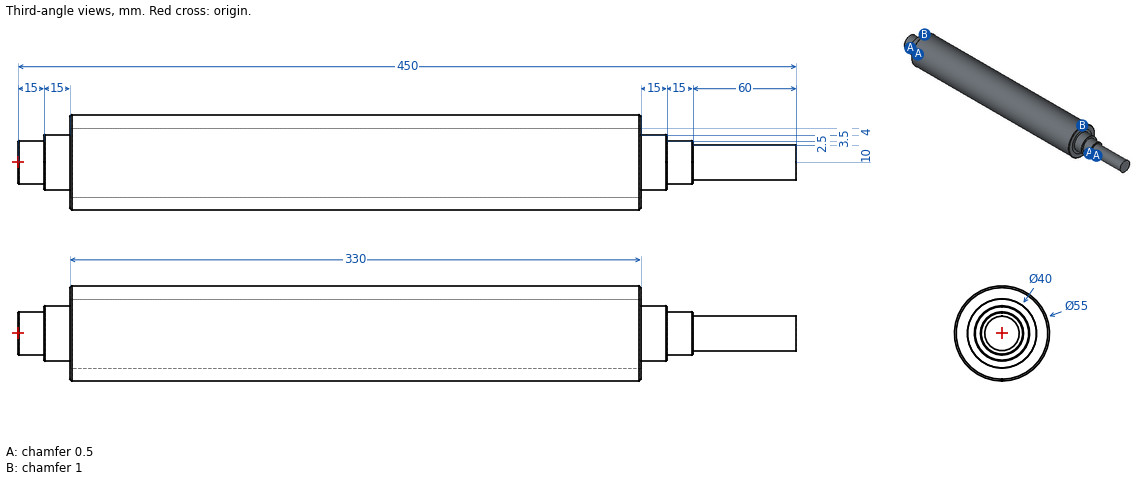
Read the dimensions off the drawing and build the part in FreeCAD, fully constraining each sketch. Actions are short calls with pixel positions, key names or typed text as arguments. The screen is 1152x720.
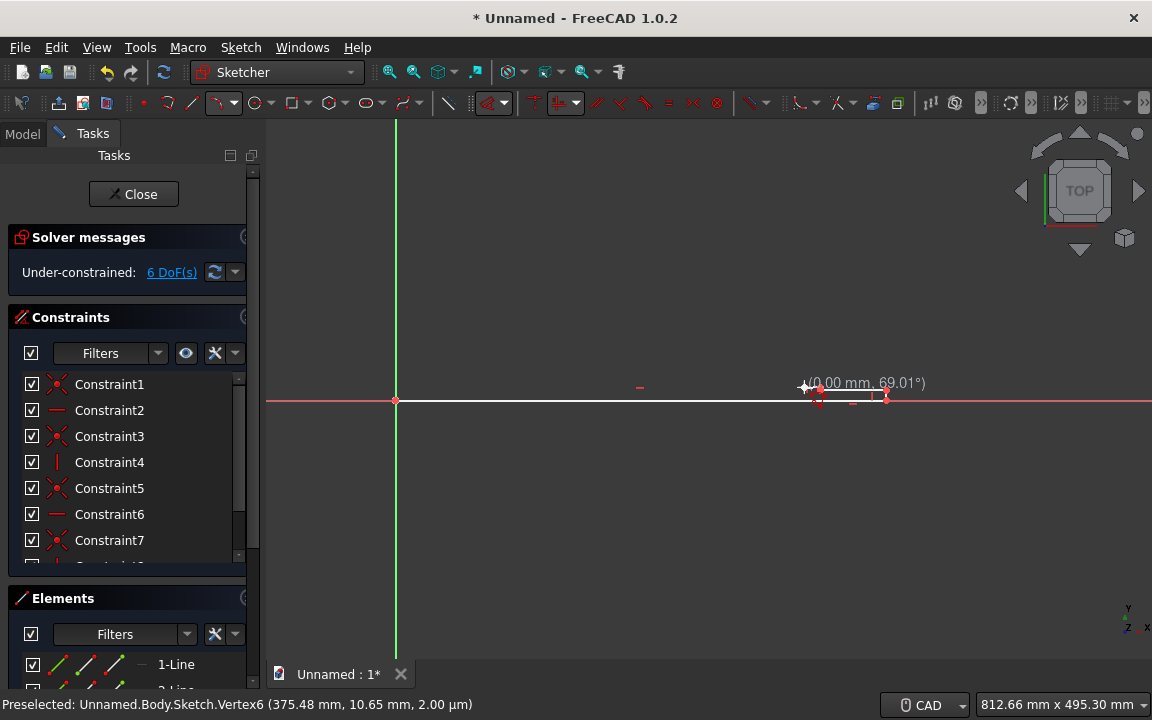
scroll(804, 383, up, 8)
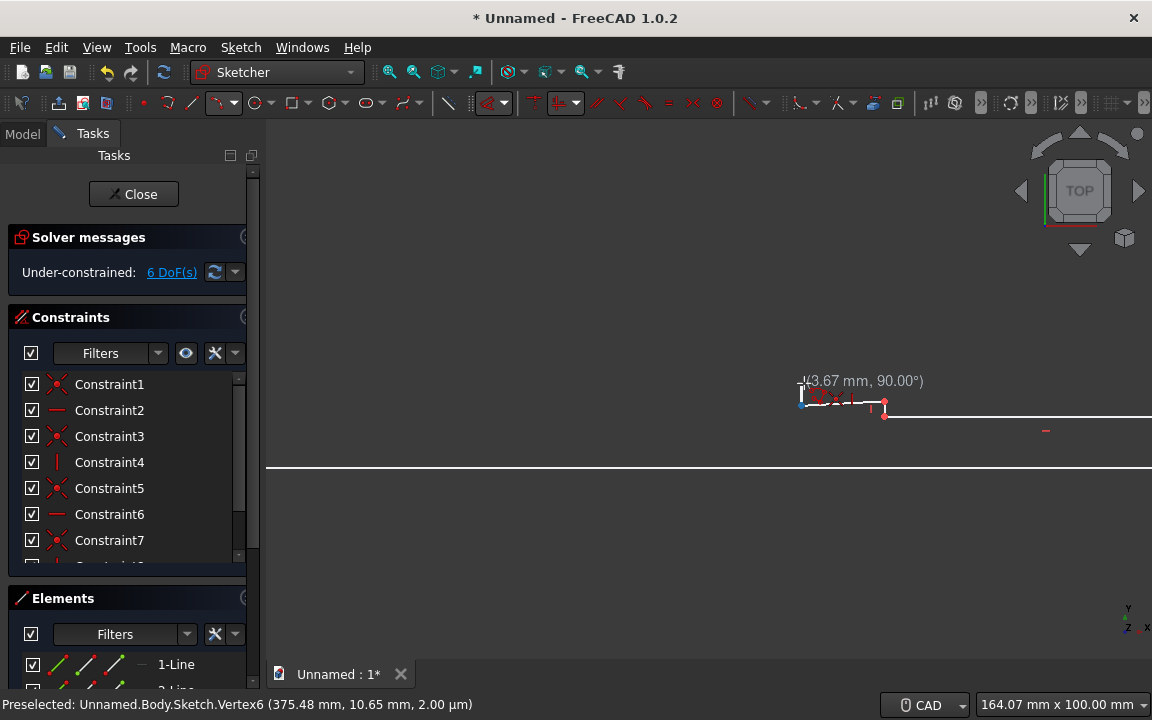
click(802, 382)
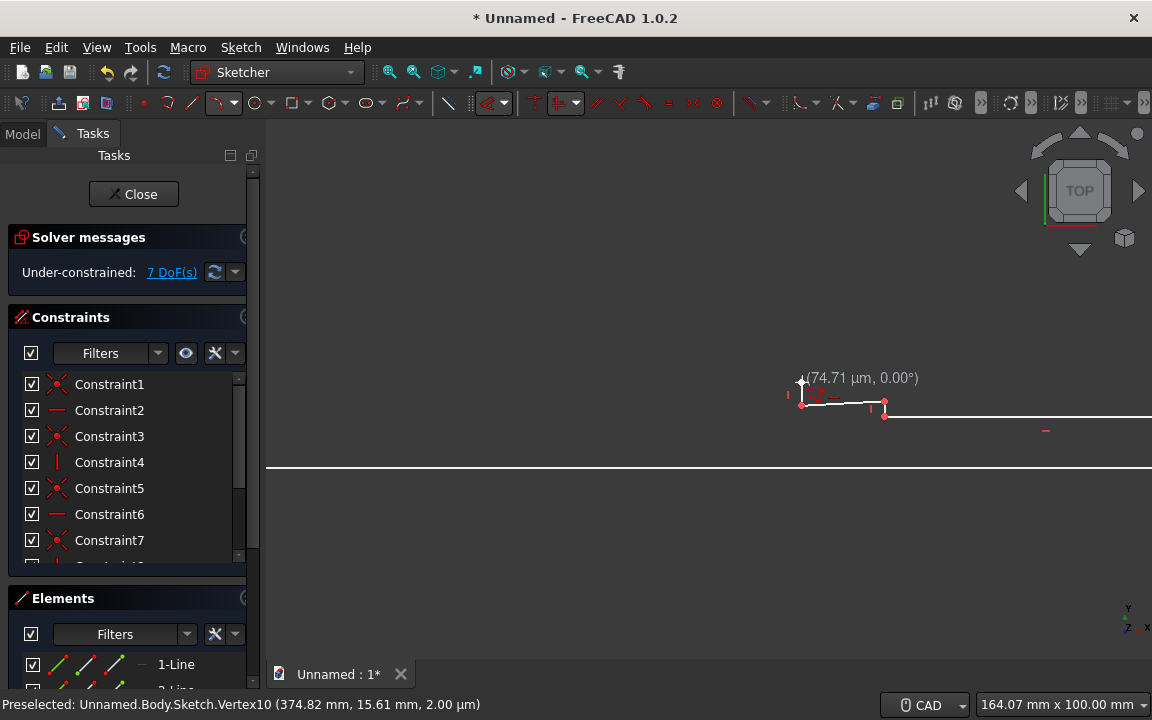
scroll(804, 383, down, 8)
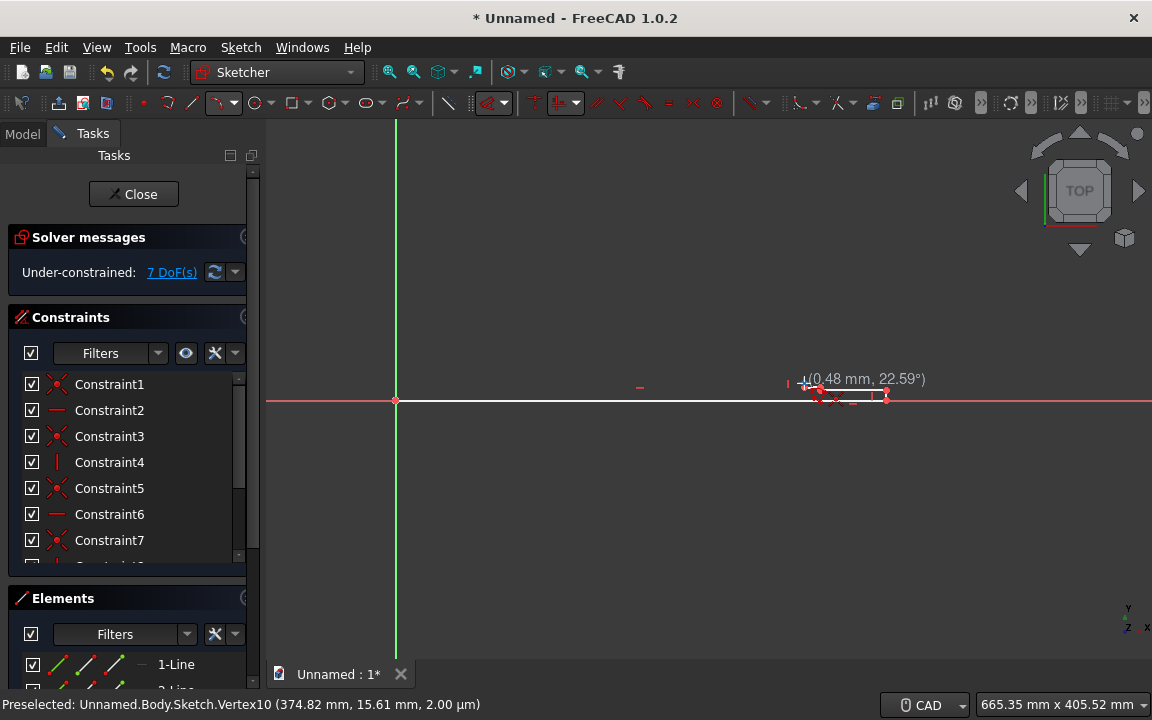
click(788, 383)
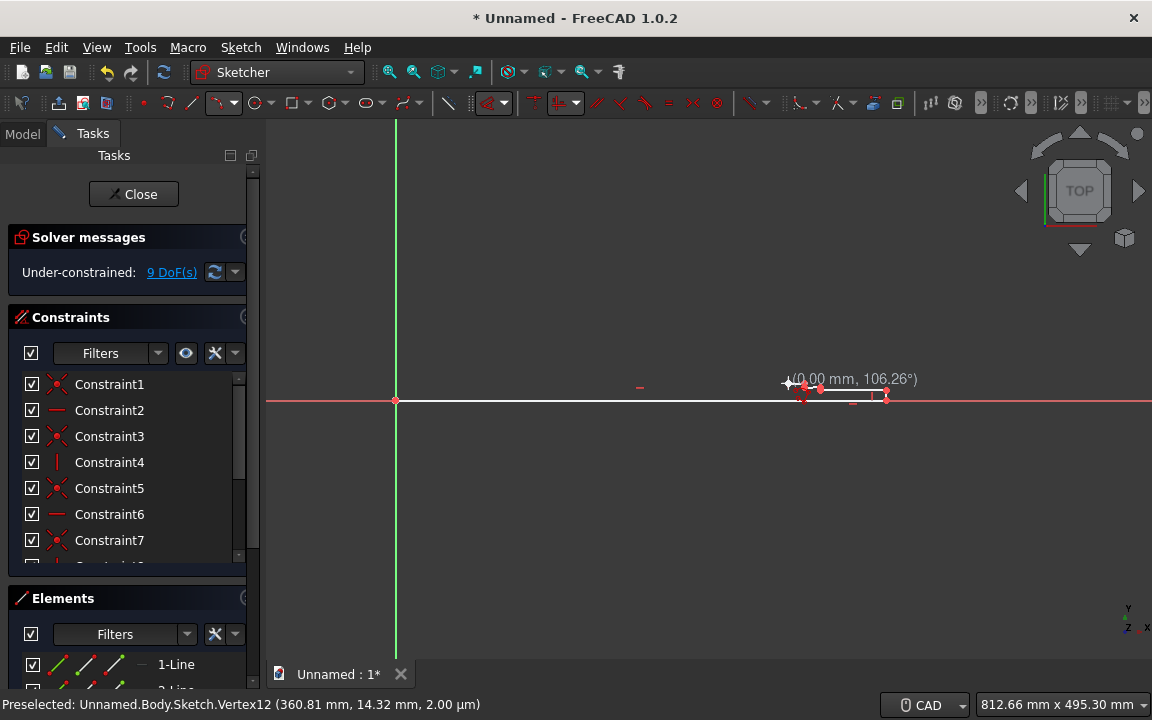
scroll(788, 379, up, 7)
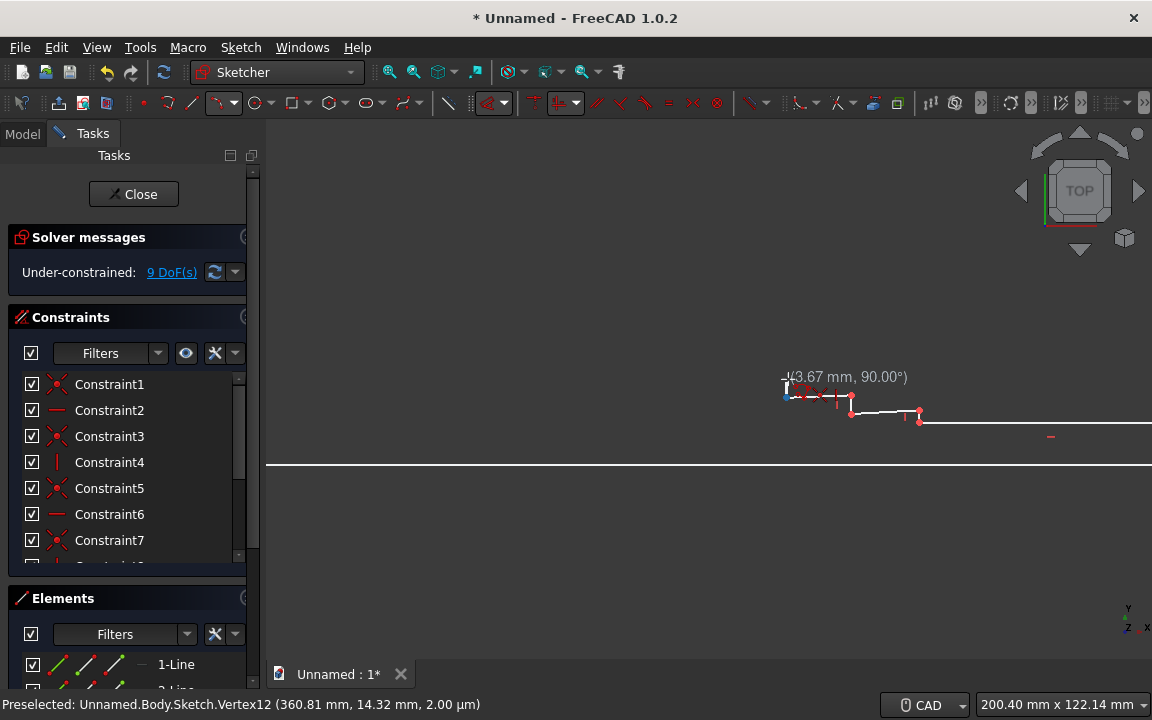
click(786, 377)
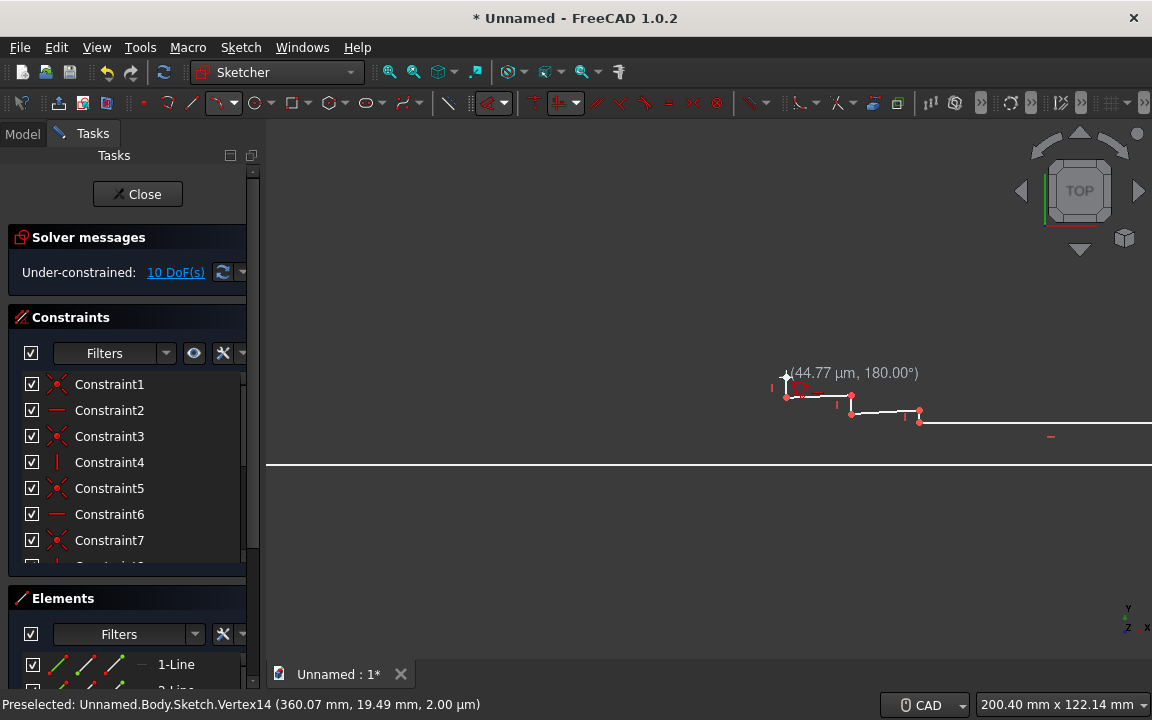
scroll(788, 379, down, 7)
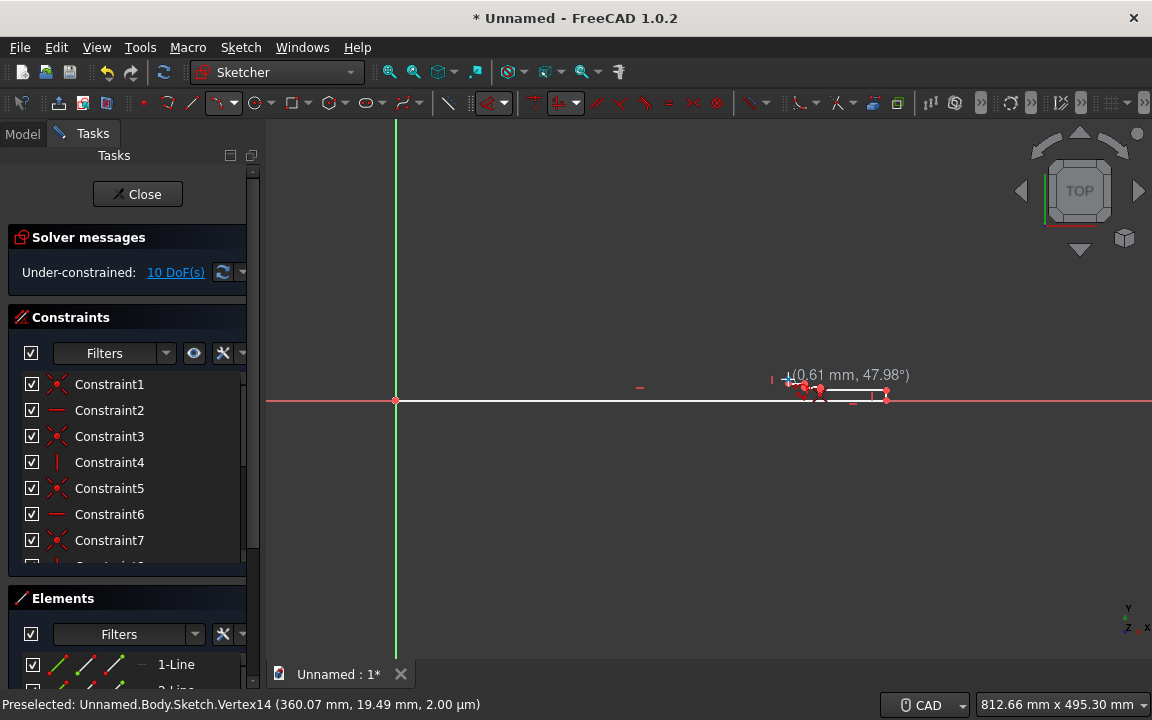
click(428, 379)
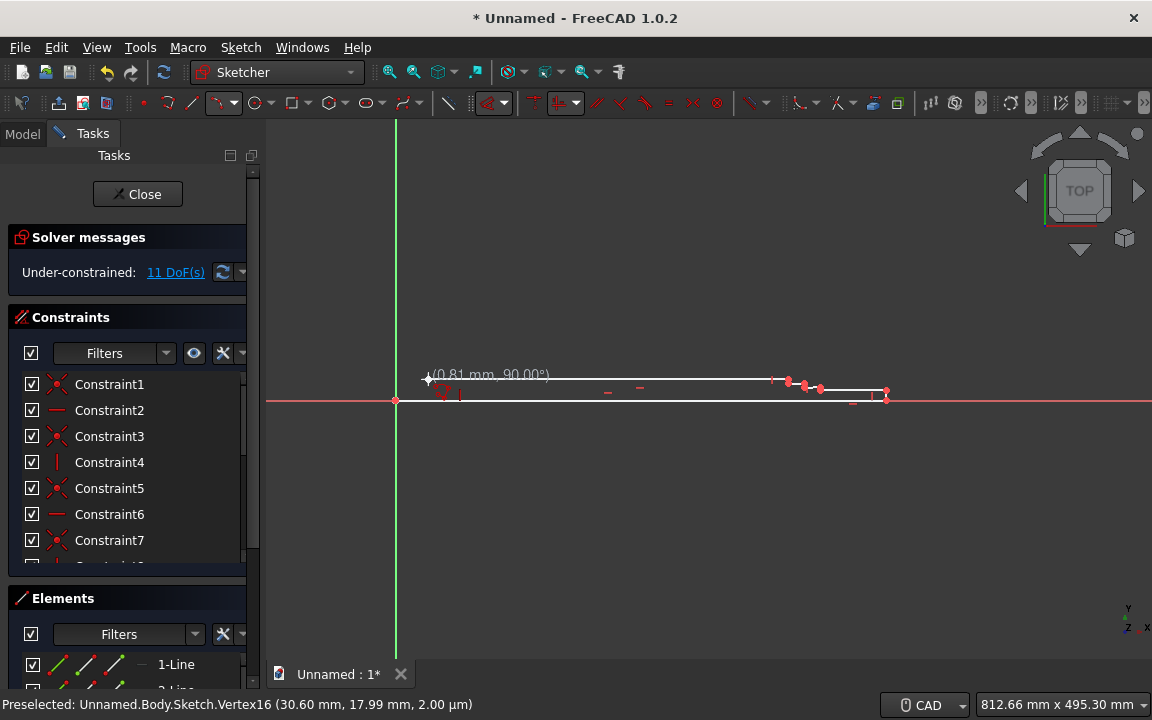
scroll(428, 383, up, 7)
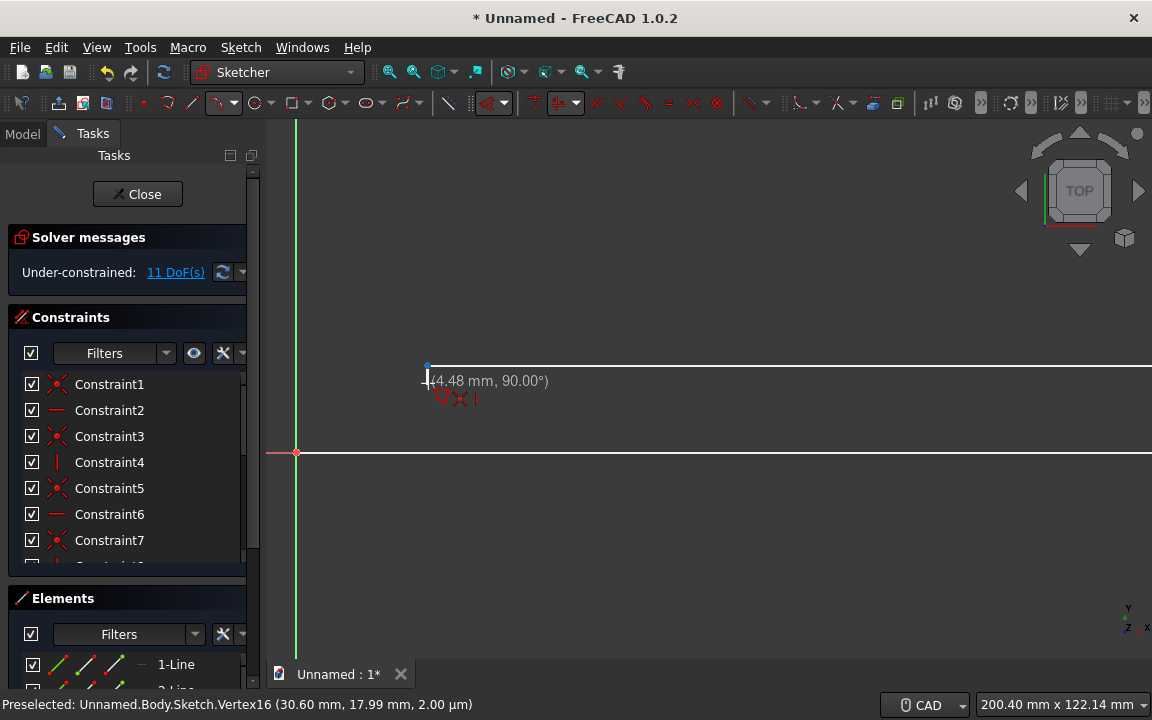
click(427, 382)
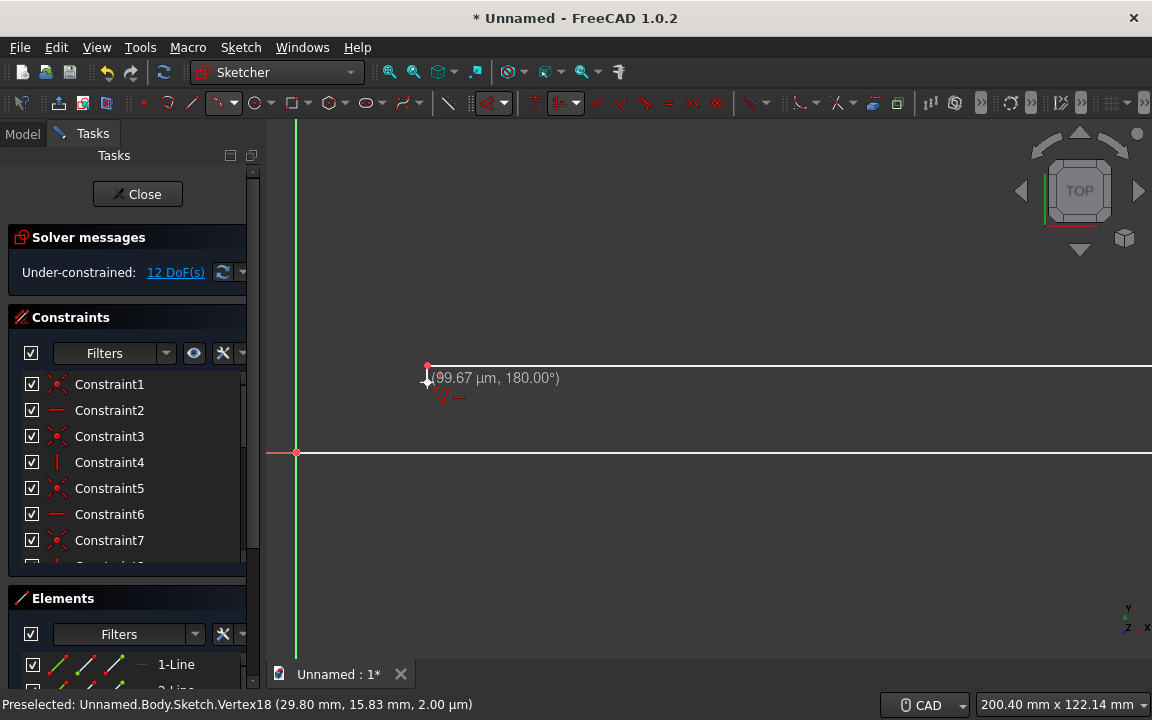
scroll(428, 383, down, 7)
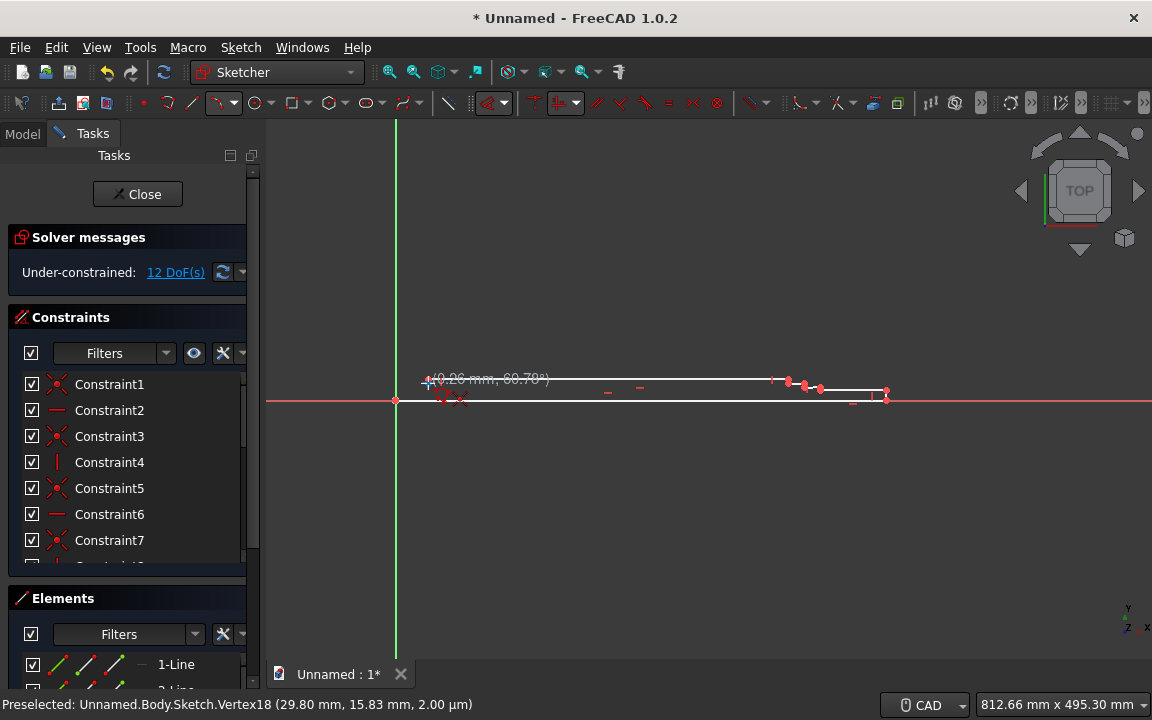
click(412, 383)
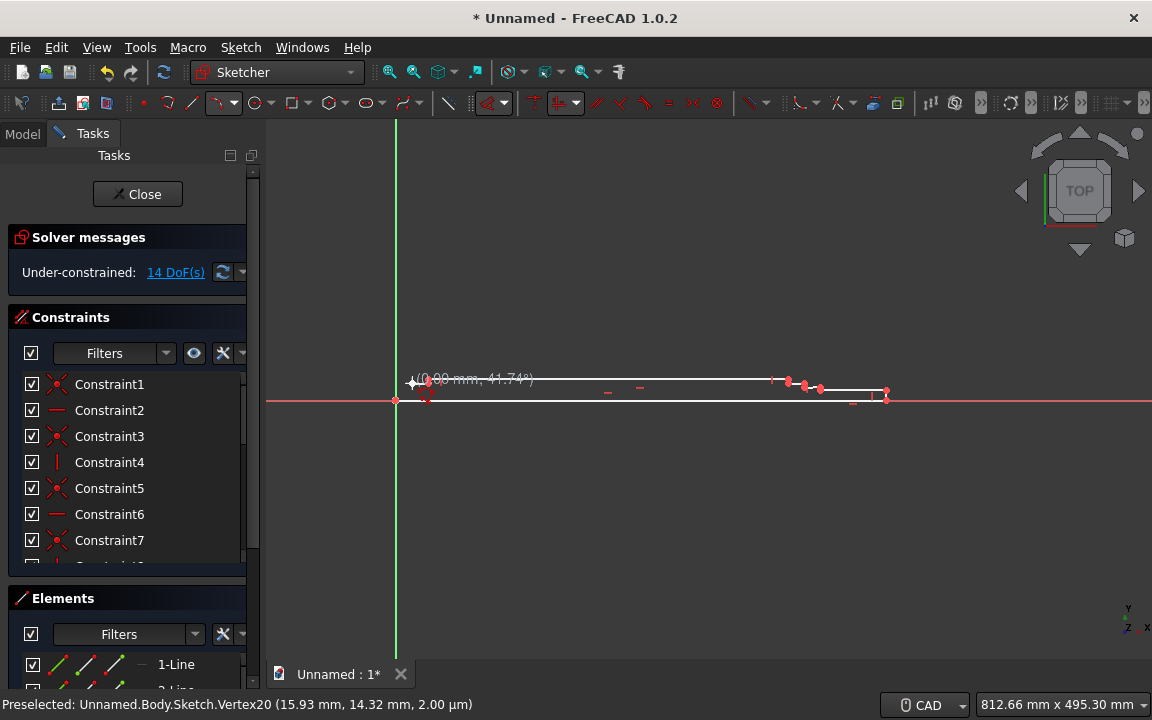
scroll(412, 387, up, 8)